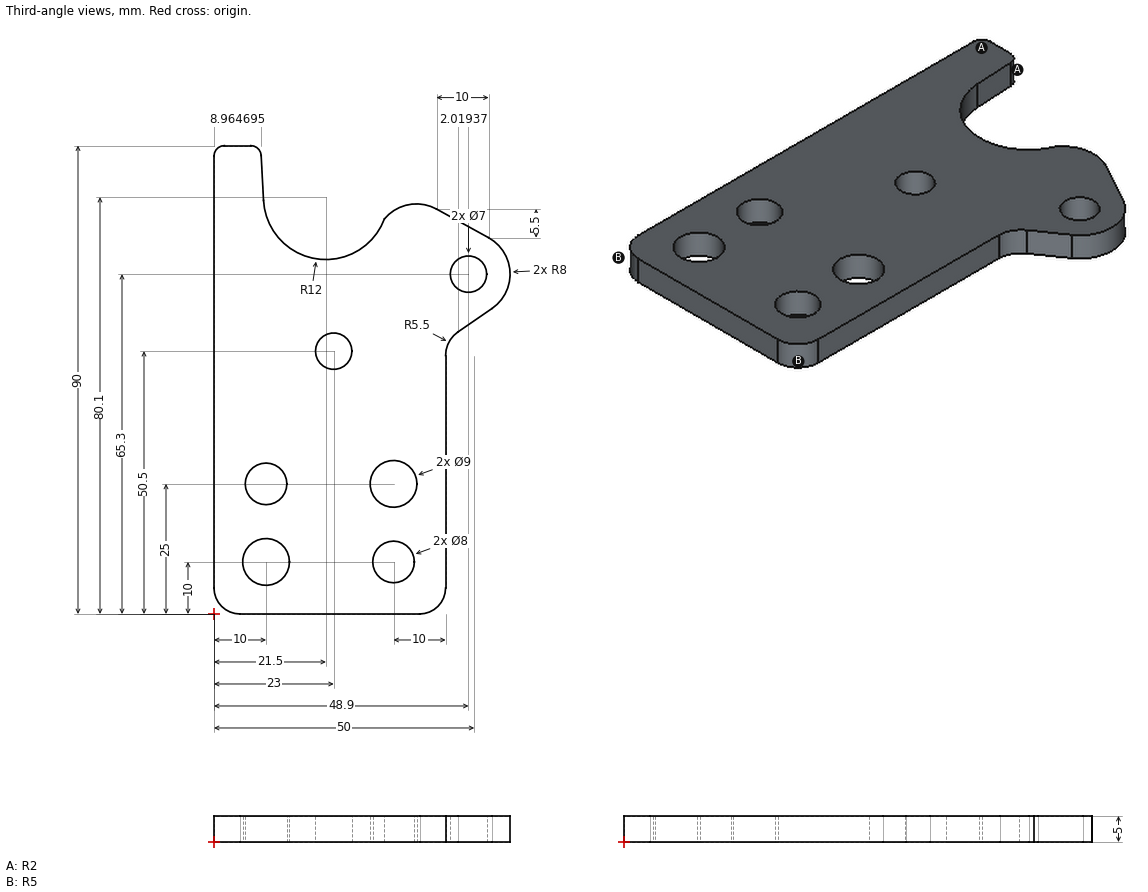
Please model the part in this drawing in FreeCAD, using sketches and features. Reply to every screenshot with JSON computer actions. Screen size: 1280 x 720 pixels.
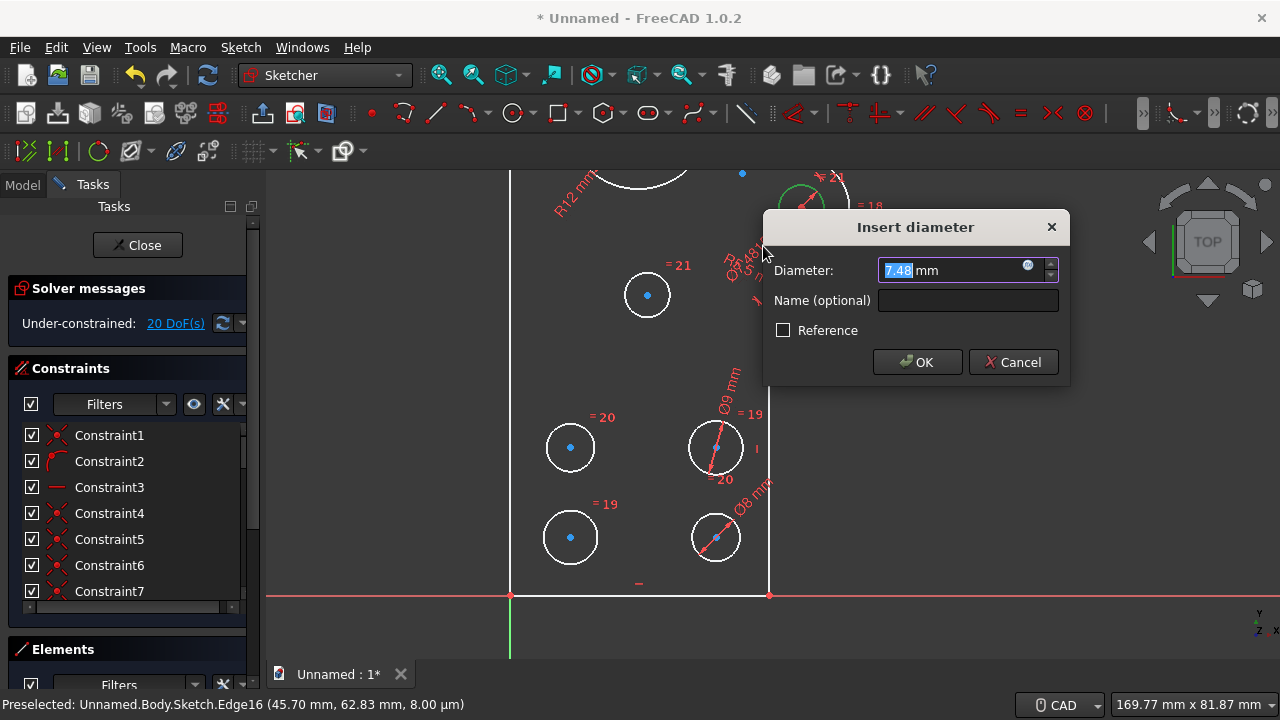
{"action": "type", "text": "7"}
{"action": "key", "text": "Return"}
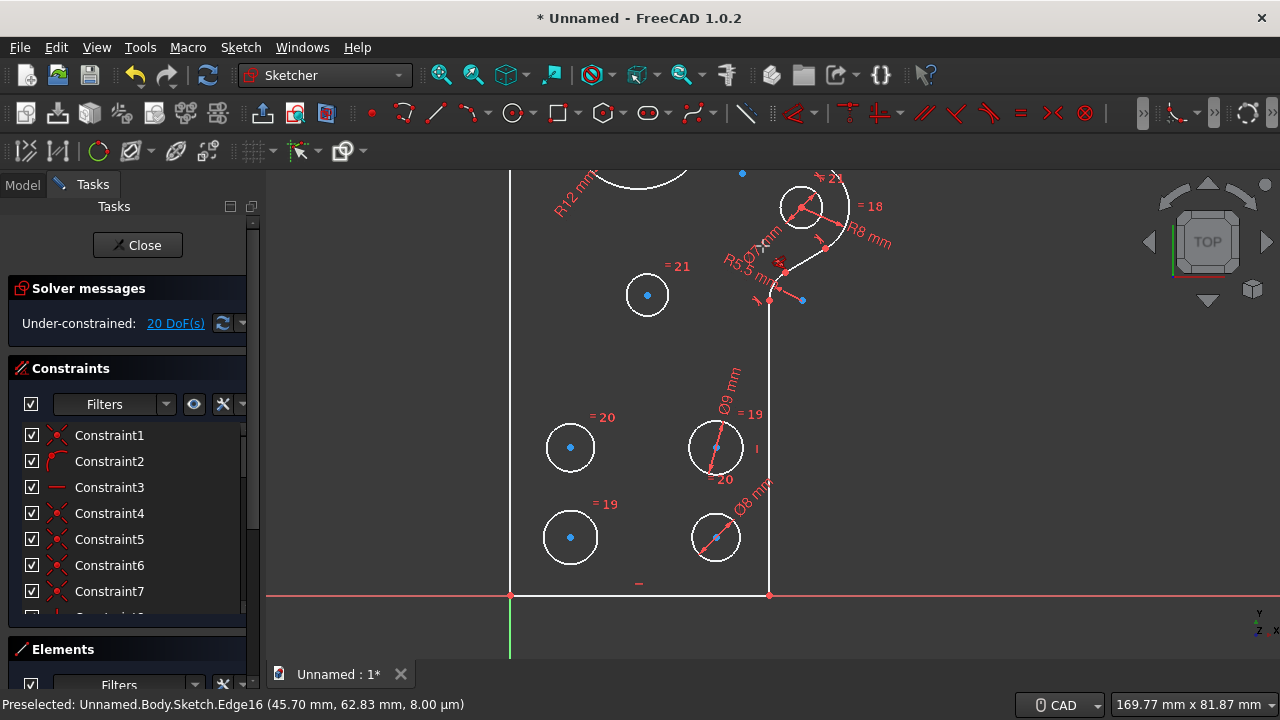
{"action": "left_click", "coordinate": [510, 222]}
{"action": "left_click", "coordinate": [476, 397]}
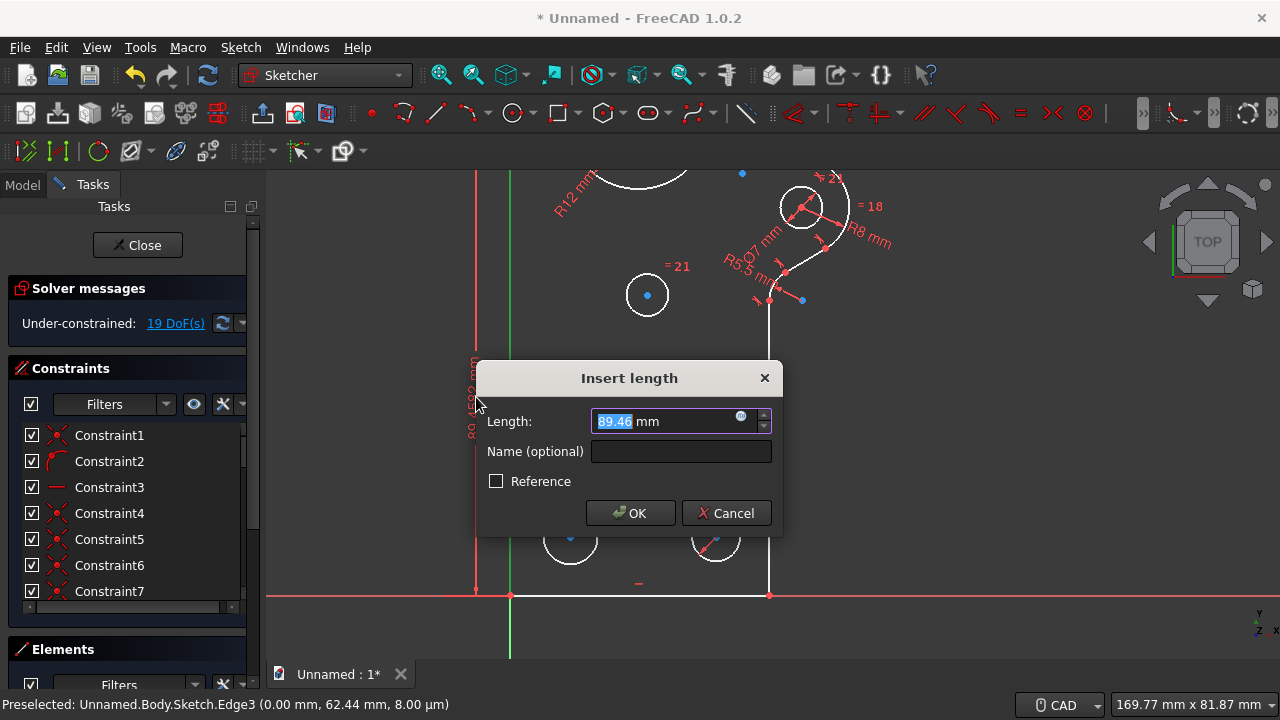
{"action": "type", "text": "90"}
{"action": "key", "text": "Return"}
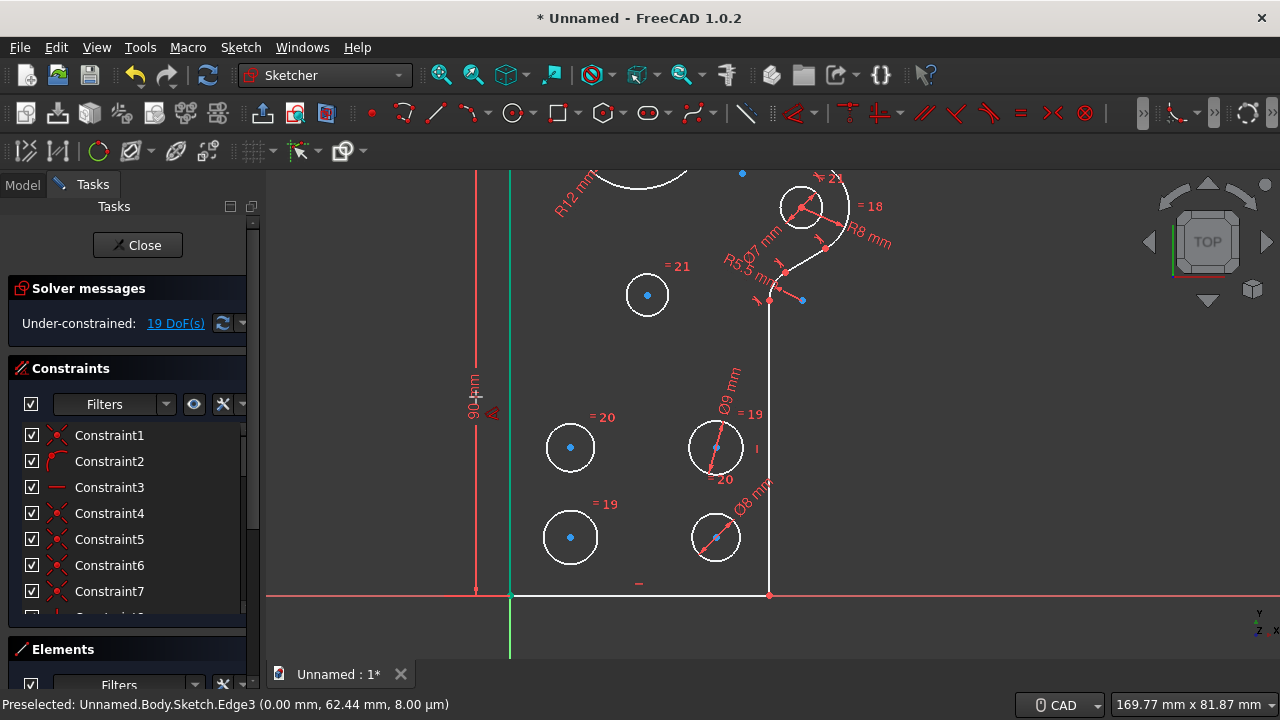
{"action": "left_click", "coordinate": [716, 537]}
{"action": "left_click", "coordinate": [476, 567]}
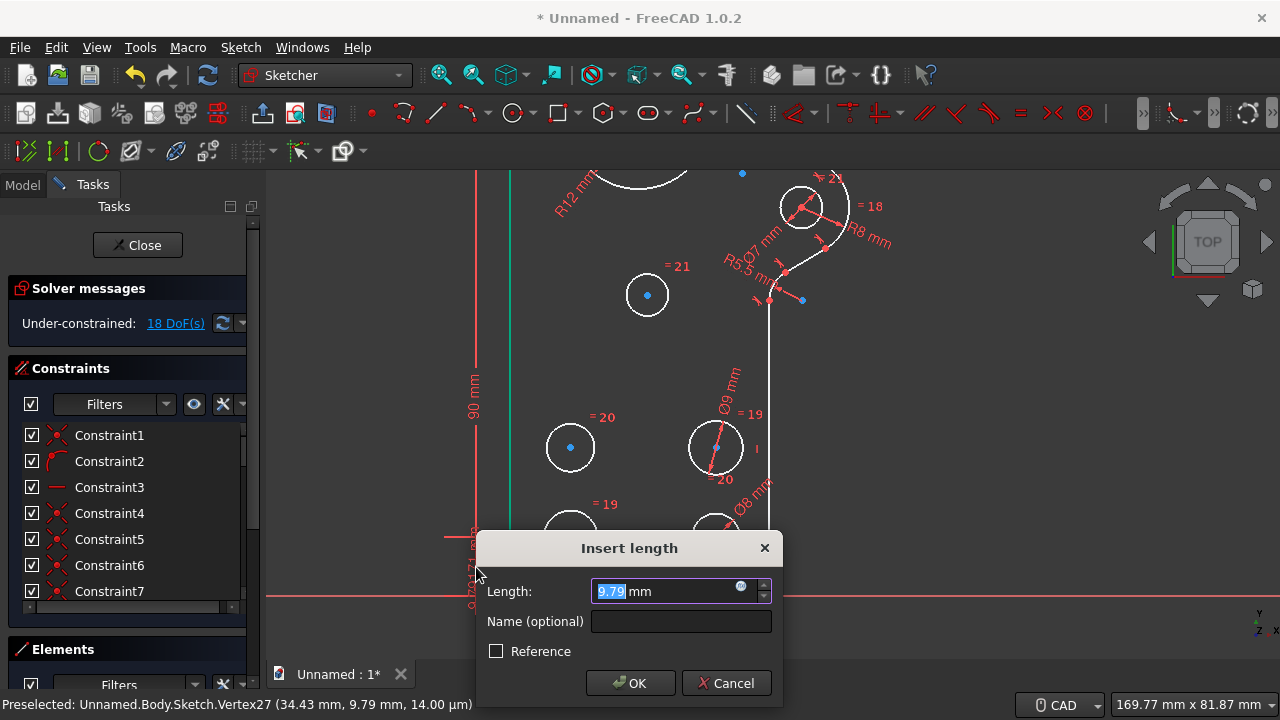
{"action": "type", "text": "10"}
{"action": "key", "text": "Return"}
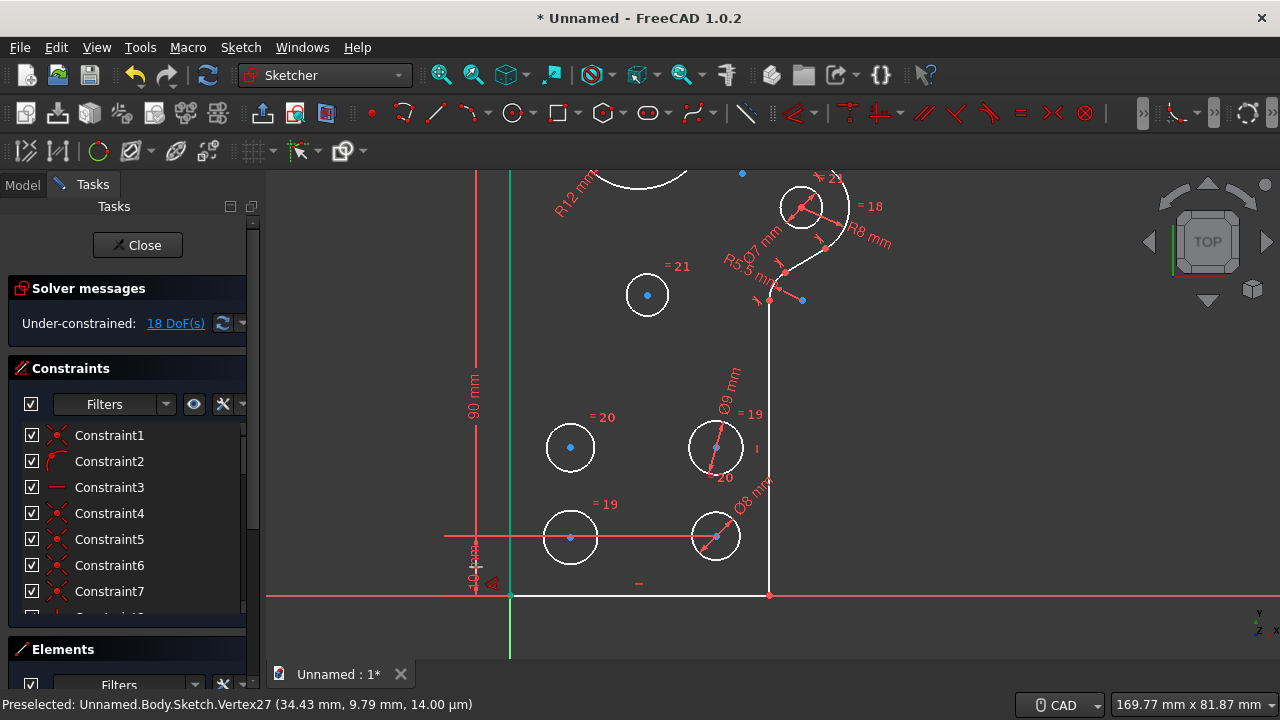
{"action": "left_click", "coordinate": [716, 448]}
{"action": "left_click", "coordinate": [476, 522]}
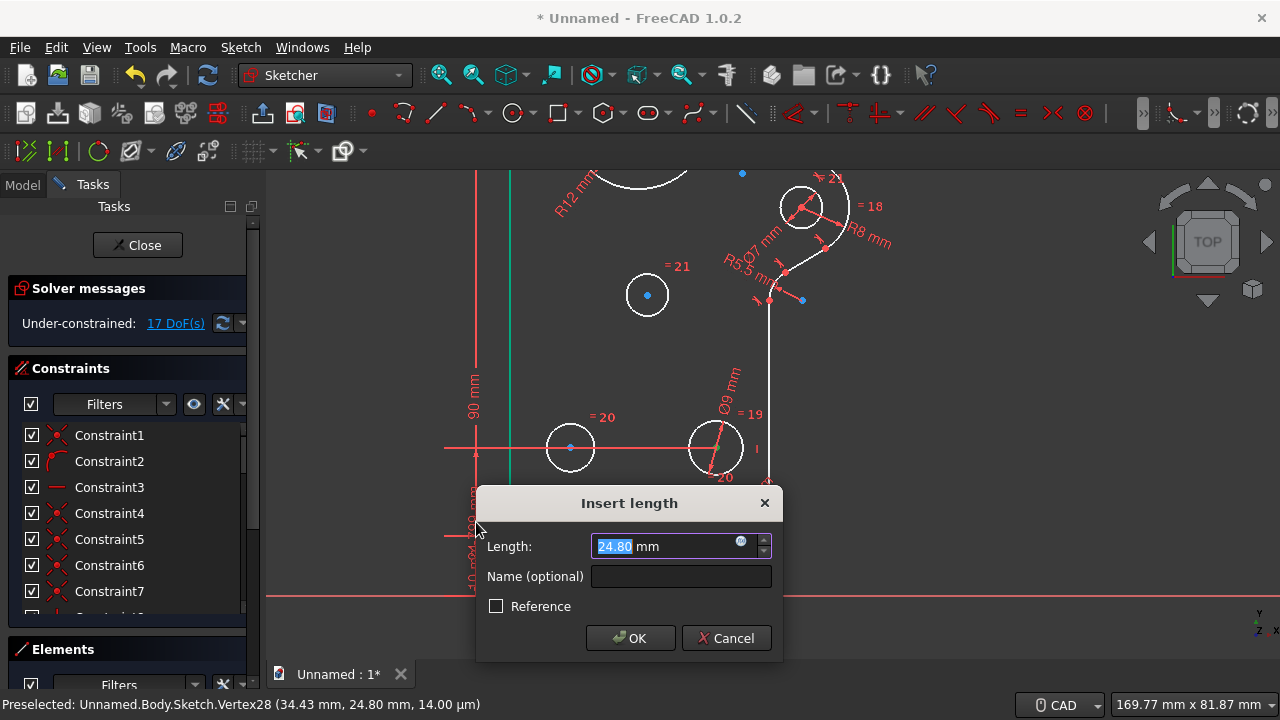
{"action": "type", "text": "25"}
{"action": "key", "text": "Return"}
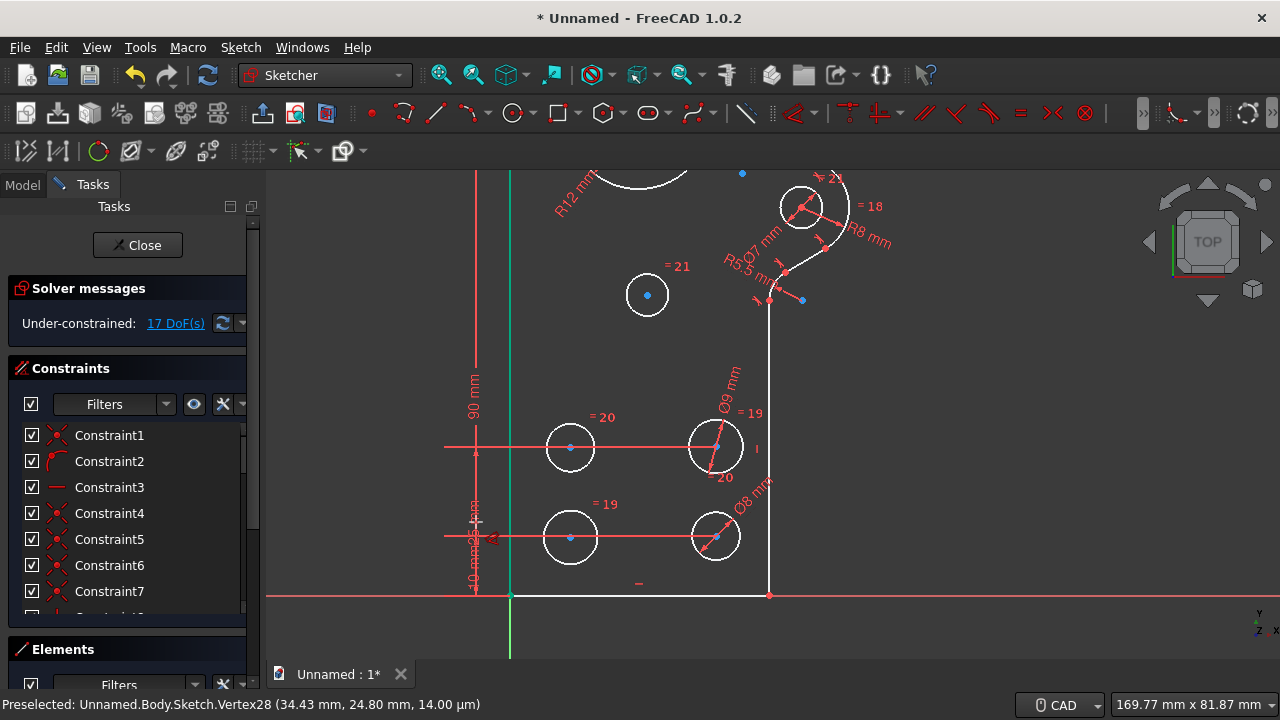
{"action": "left_click", "coordinate": [571, 537]}
{"action": "left_click", "coordinate": [540, 630]}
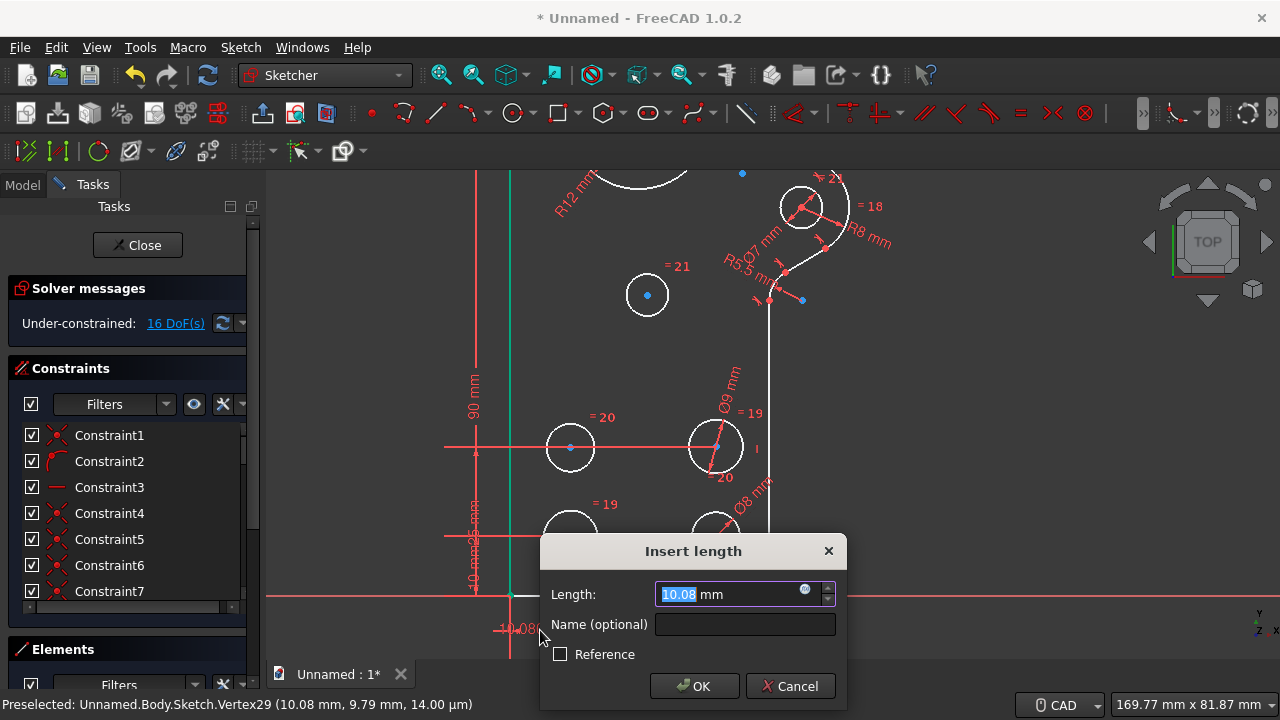
{"action": "type", "text": "10"}
{"action": "key", "text": "Return"}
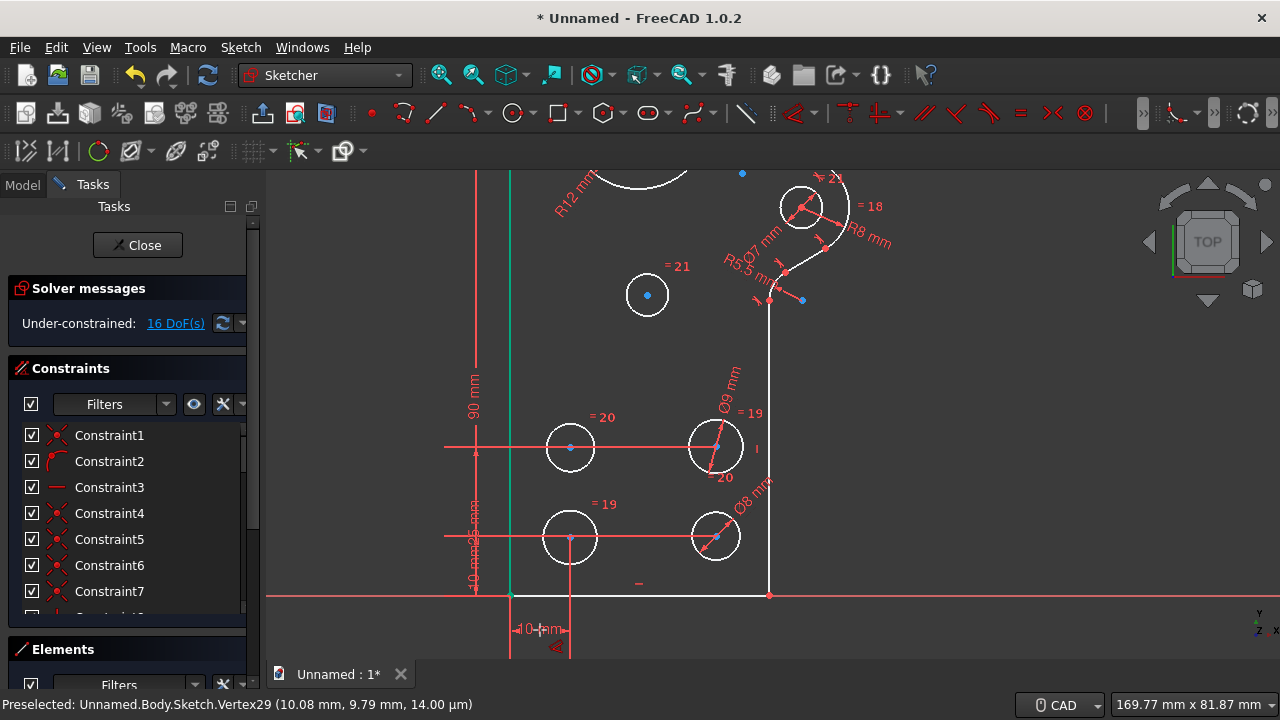
{"action": "left_click", "coordinate": [570, 537]}
{"action": "left_click", "coordinate": [476, 546]}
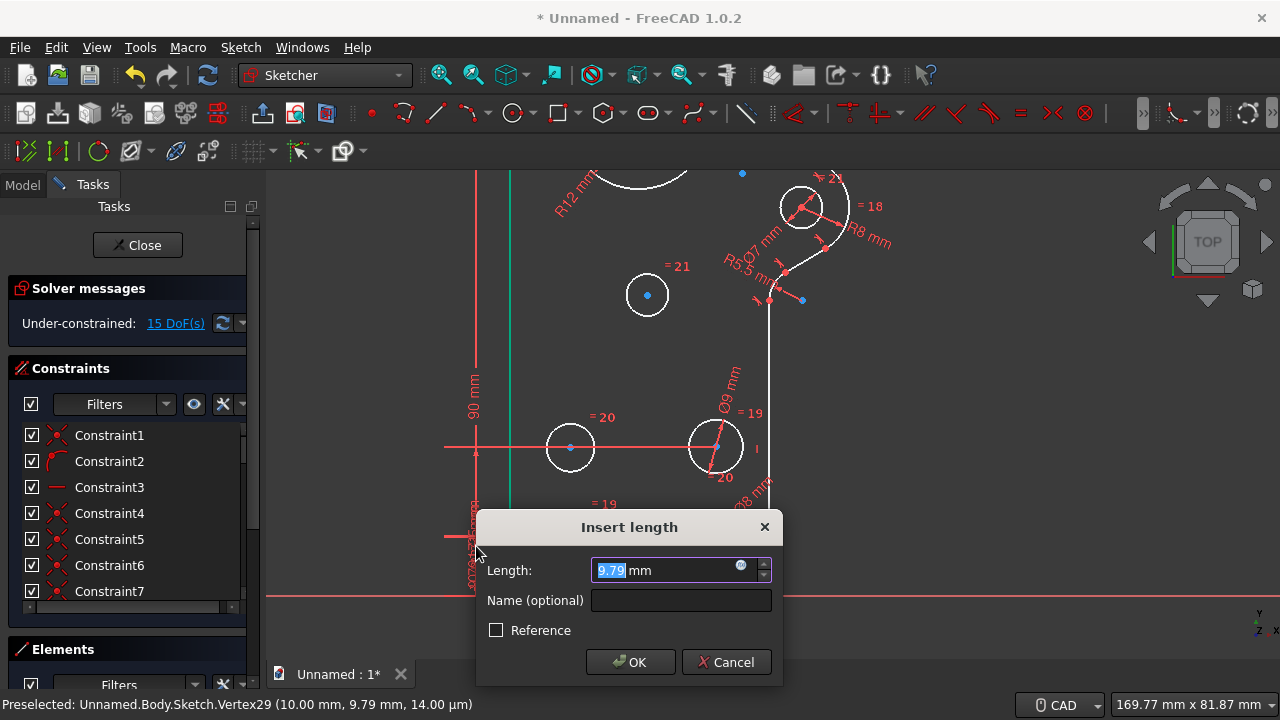
{"action": "type", "text": "10"}
{"action": "key", "text": "Return"}